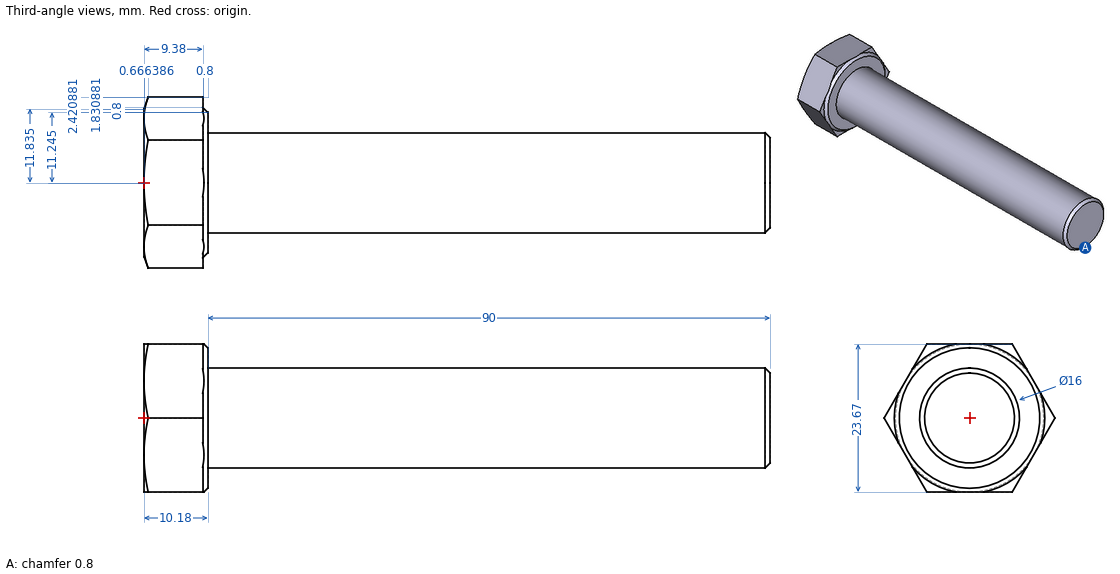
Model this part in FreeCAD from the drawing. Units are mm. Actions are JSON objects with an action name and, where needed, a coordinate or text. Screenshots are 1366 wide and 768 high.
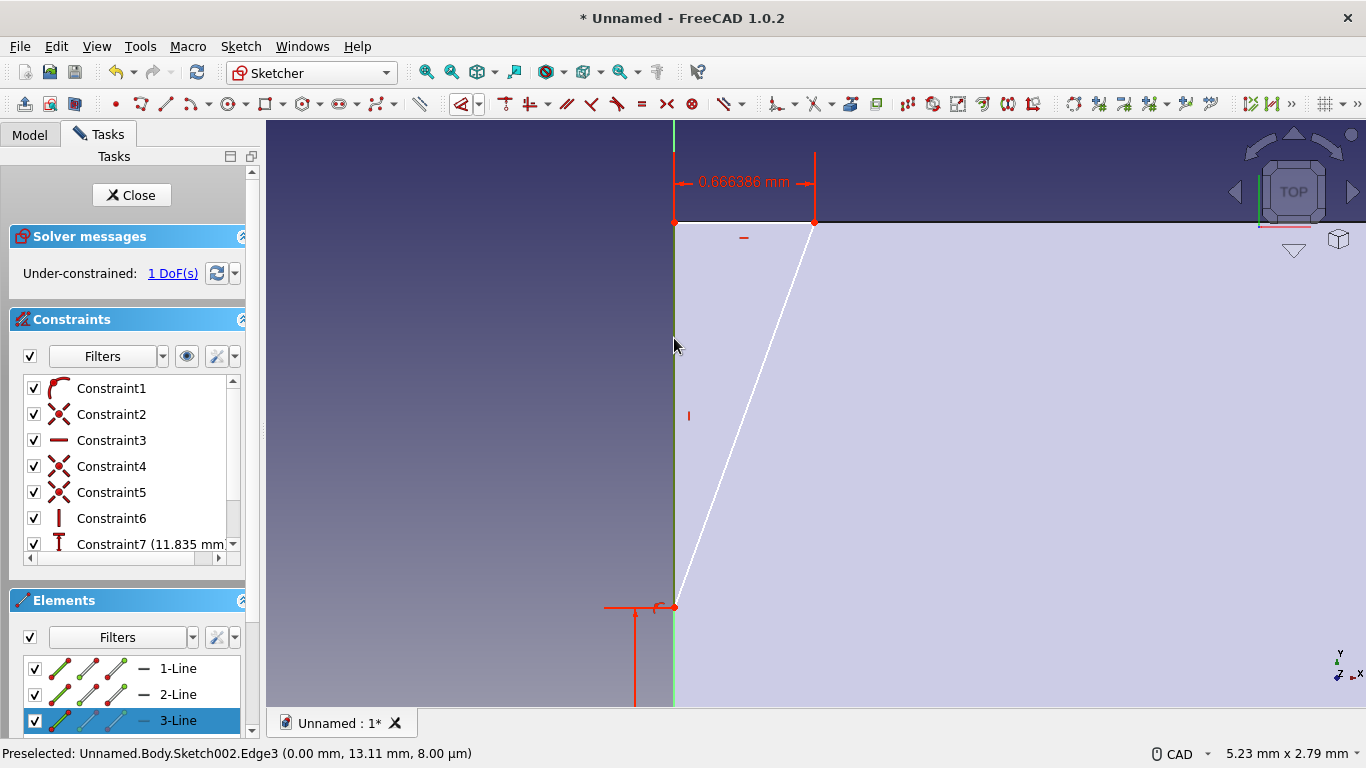
{"action": "key", "text": "i"}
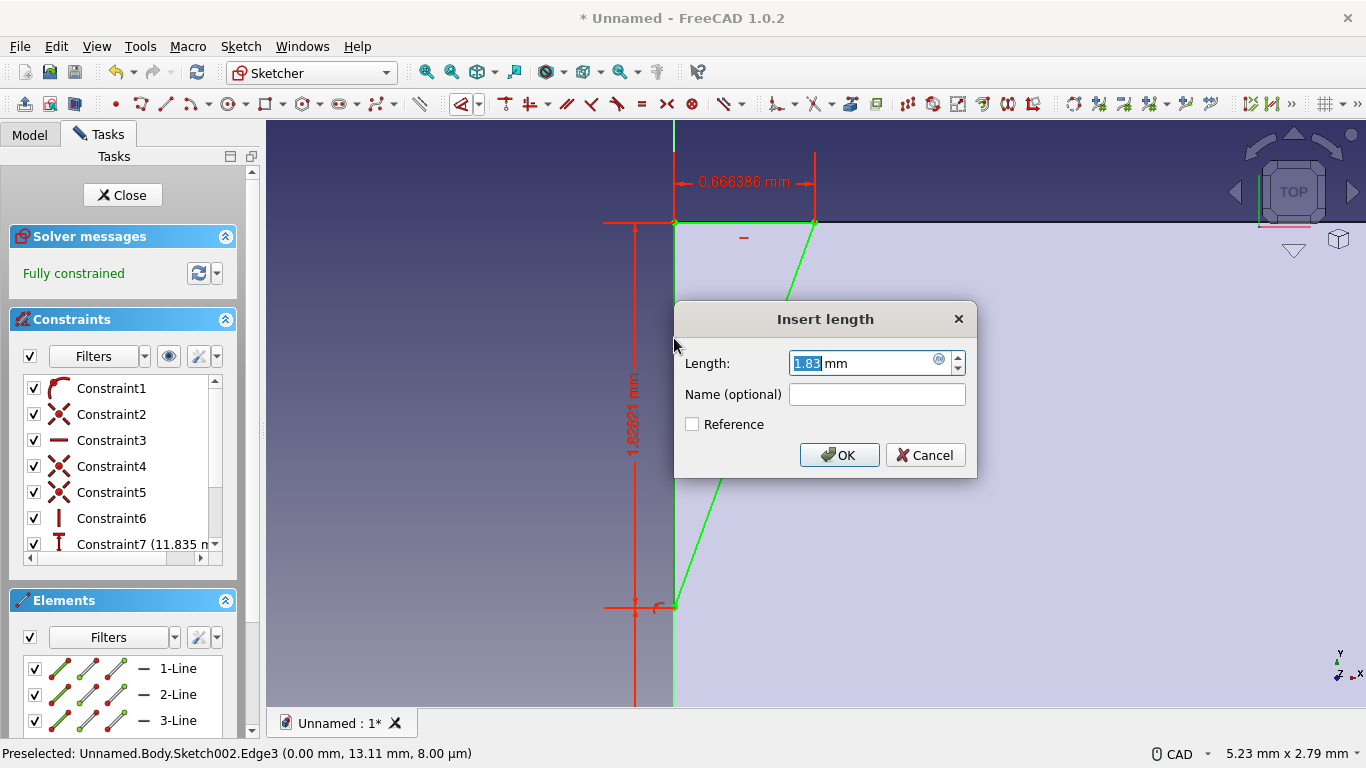
{"action": "type", "text": "1.830881"}
{"action": "key", "text": "Return"}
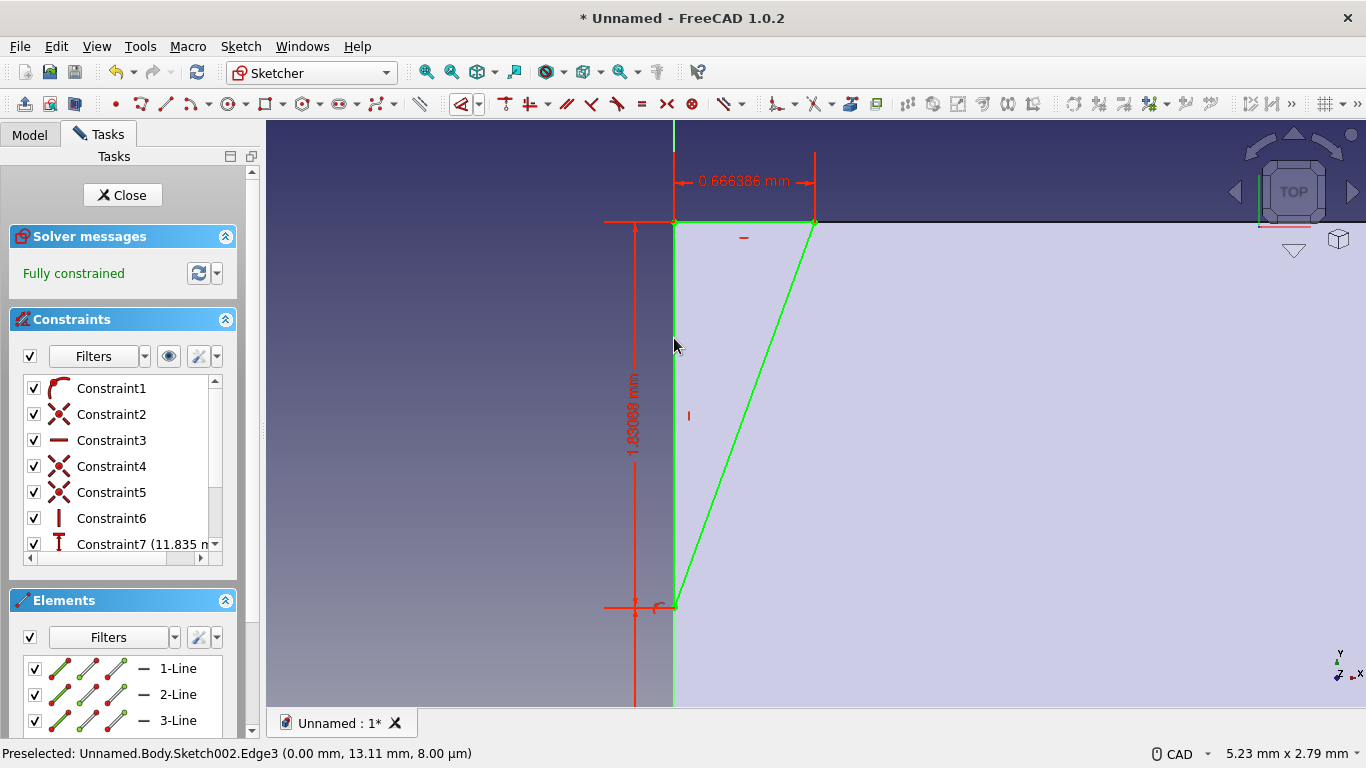
{"action": "left_click", "coordinate": [123, 195]}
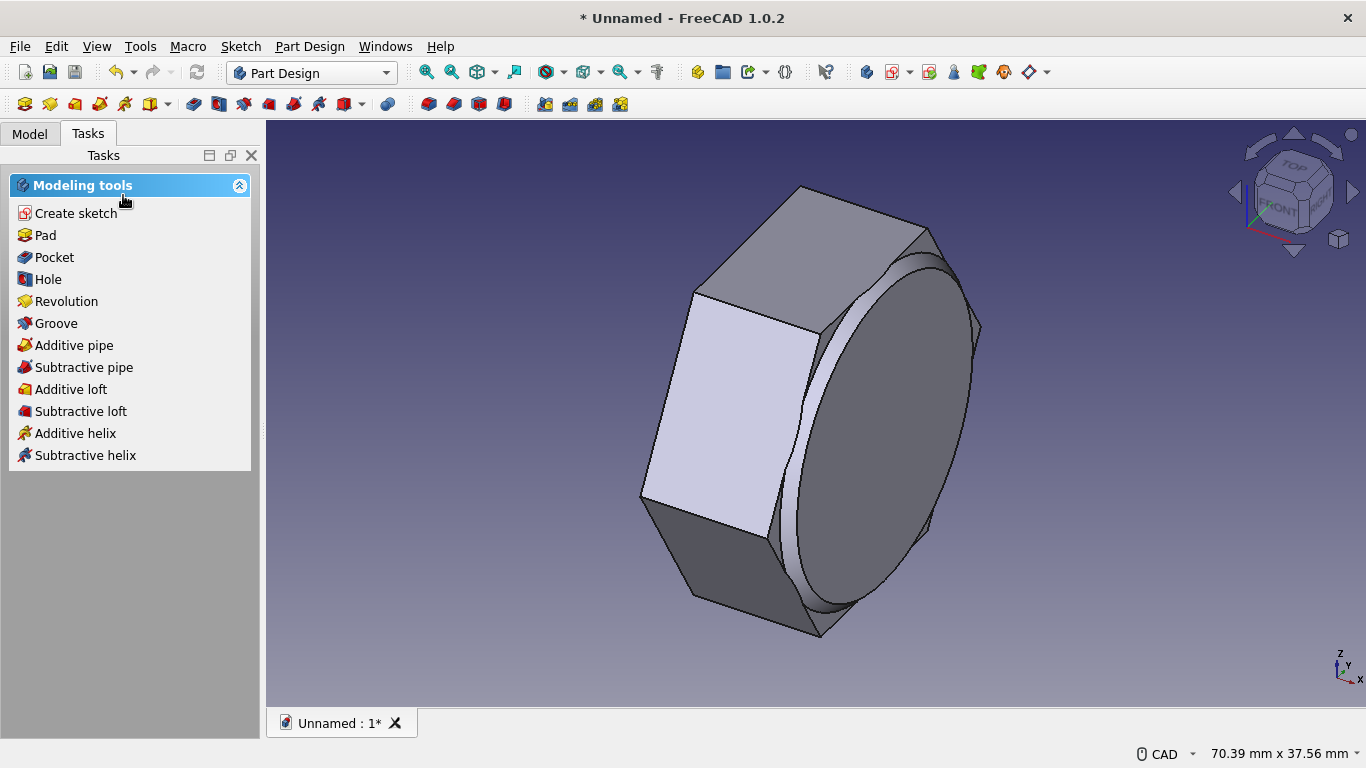
{"action": "left_click", "coordinate": [244, 104]}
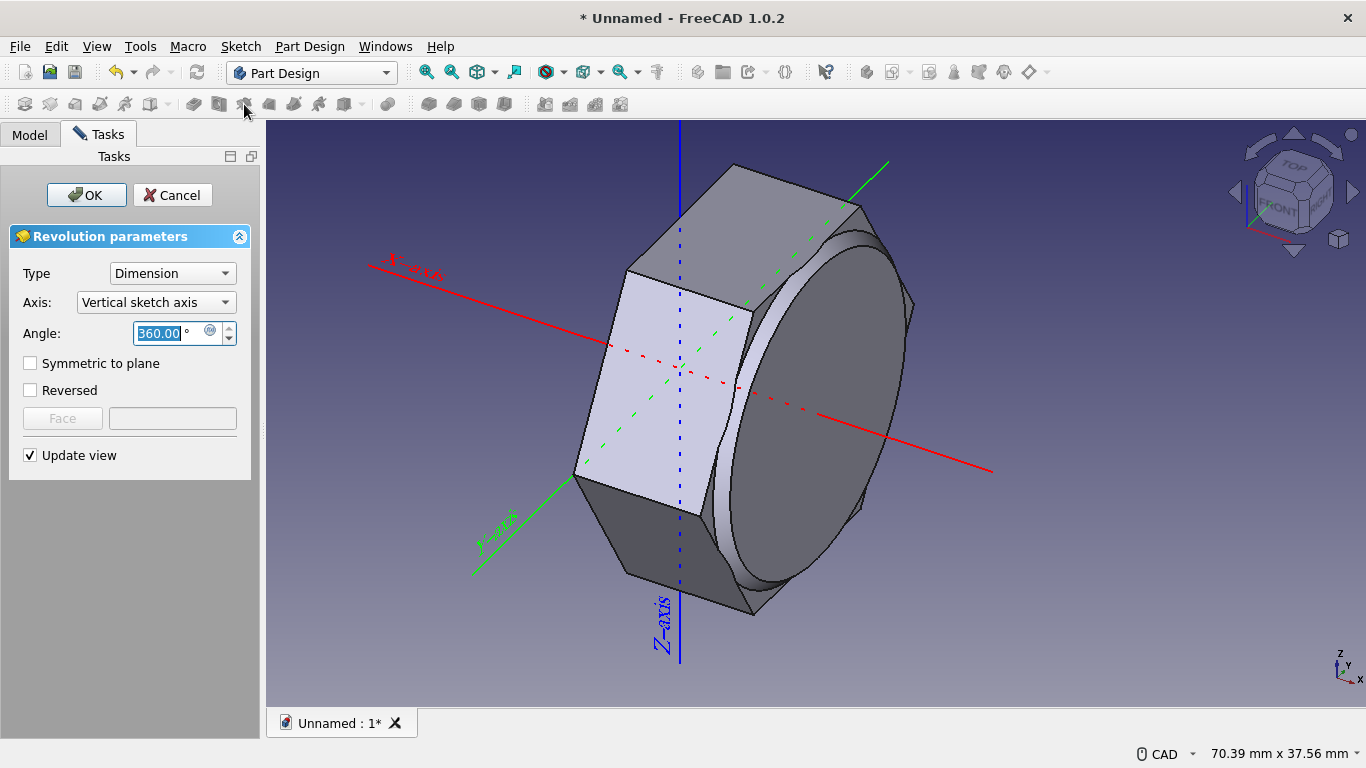
{"action": "left_click", "coordinate": [157, 302]}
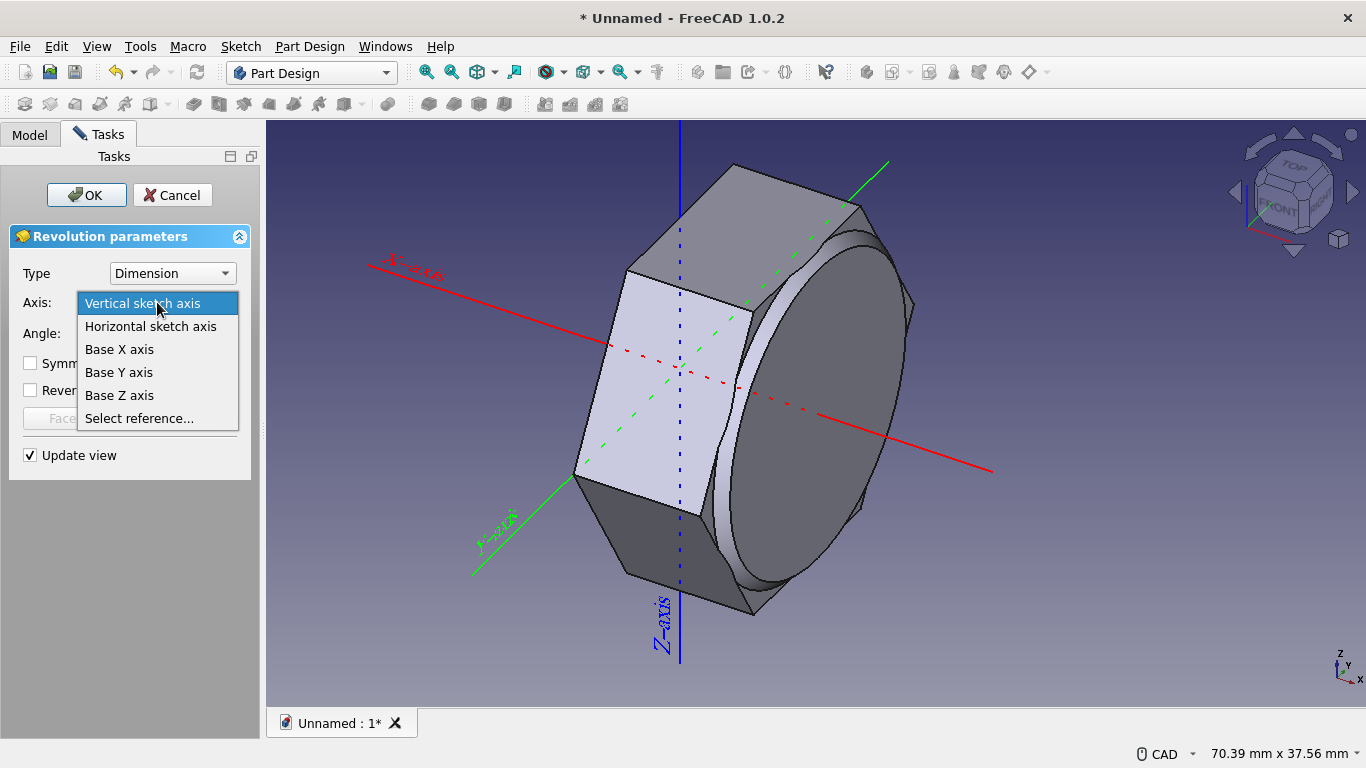
{"action": "left_click", "coordinate": [156, 326]}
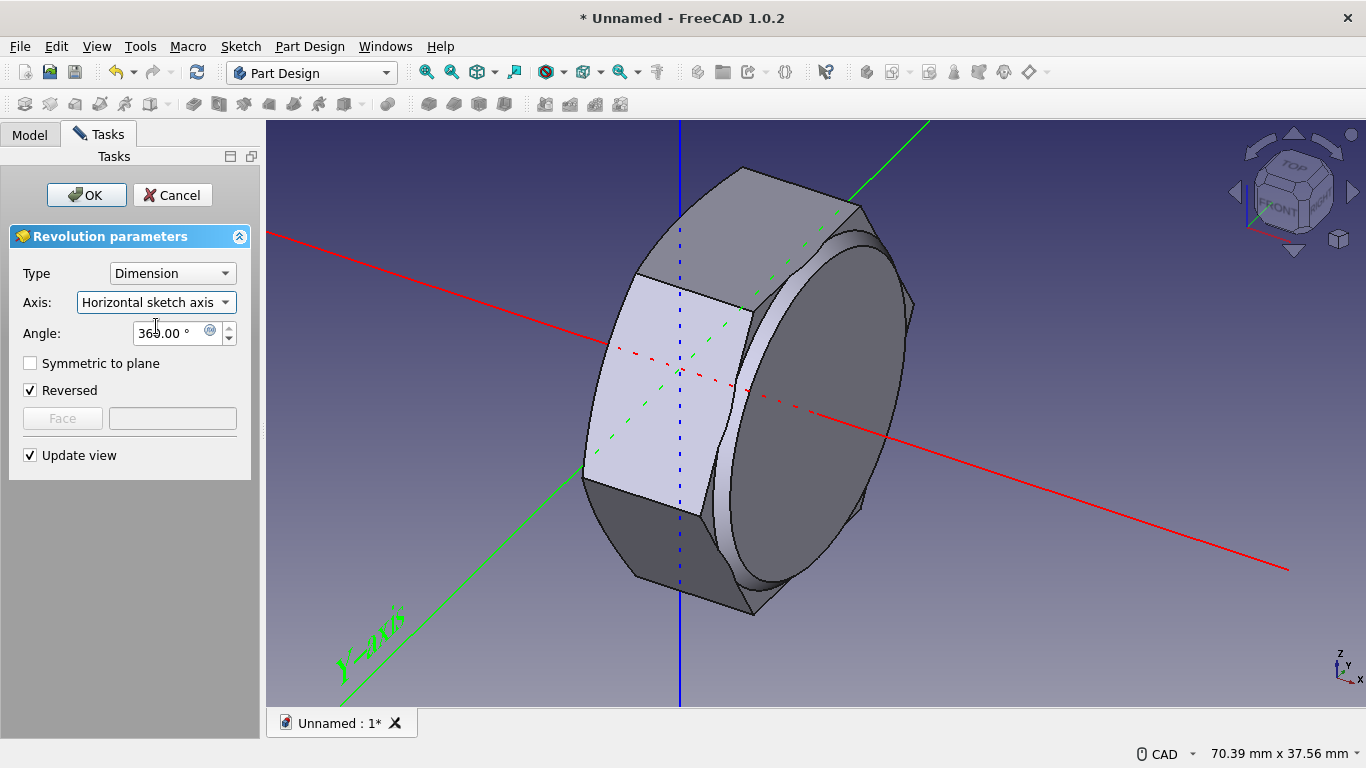
{"action": "left_click", "coordinate": [87, 195]}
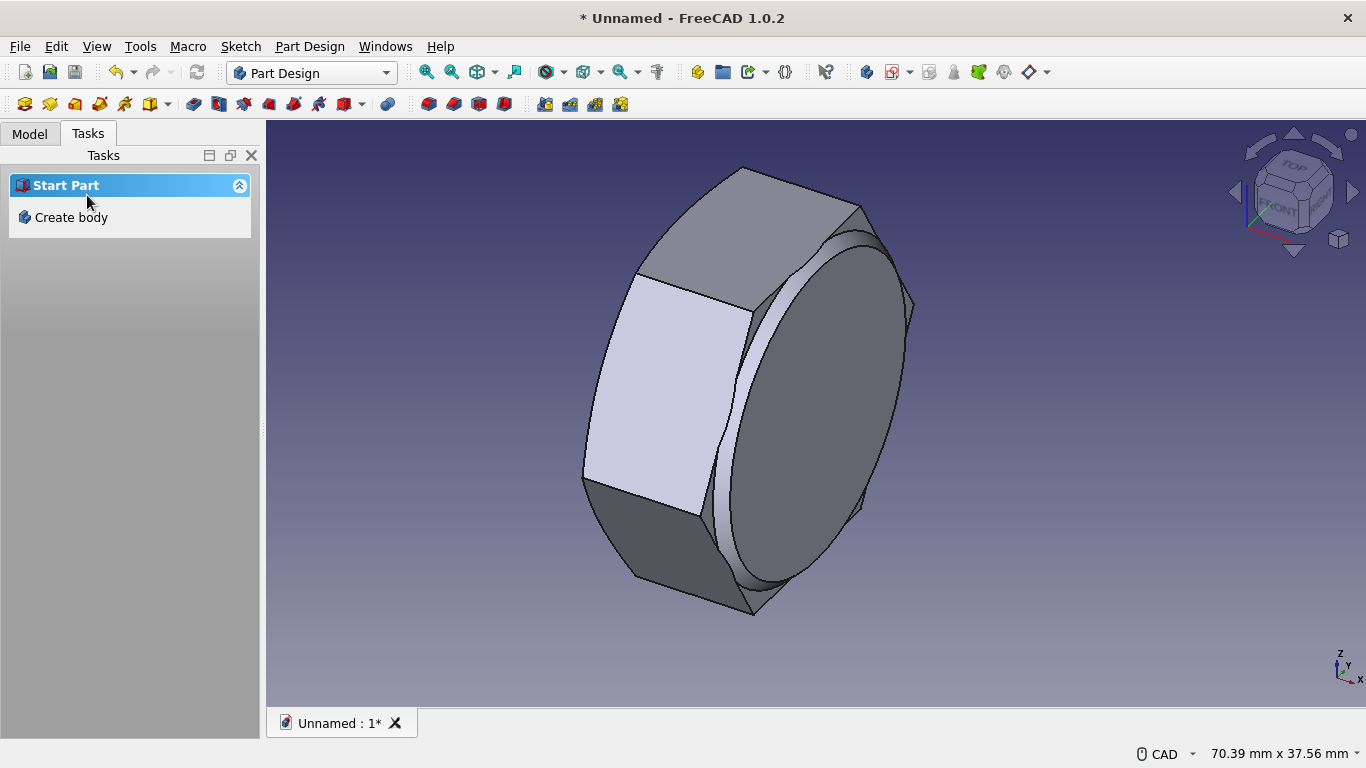
{"action": "key", "text": "v f"}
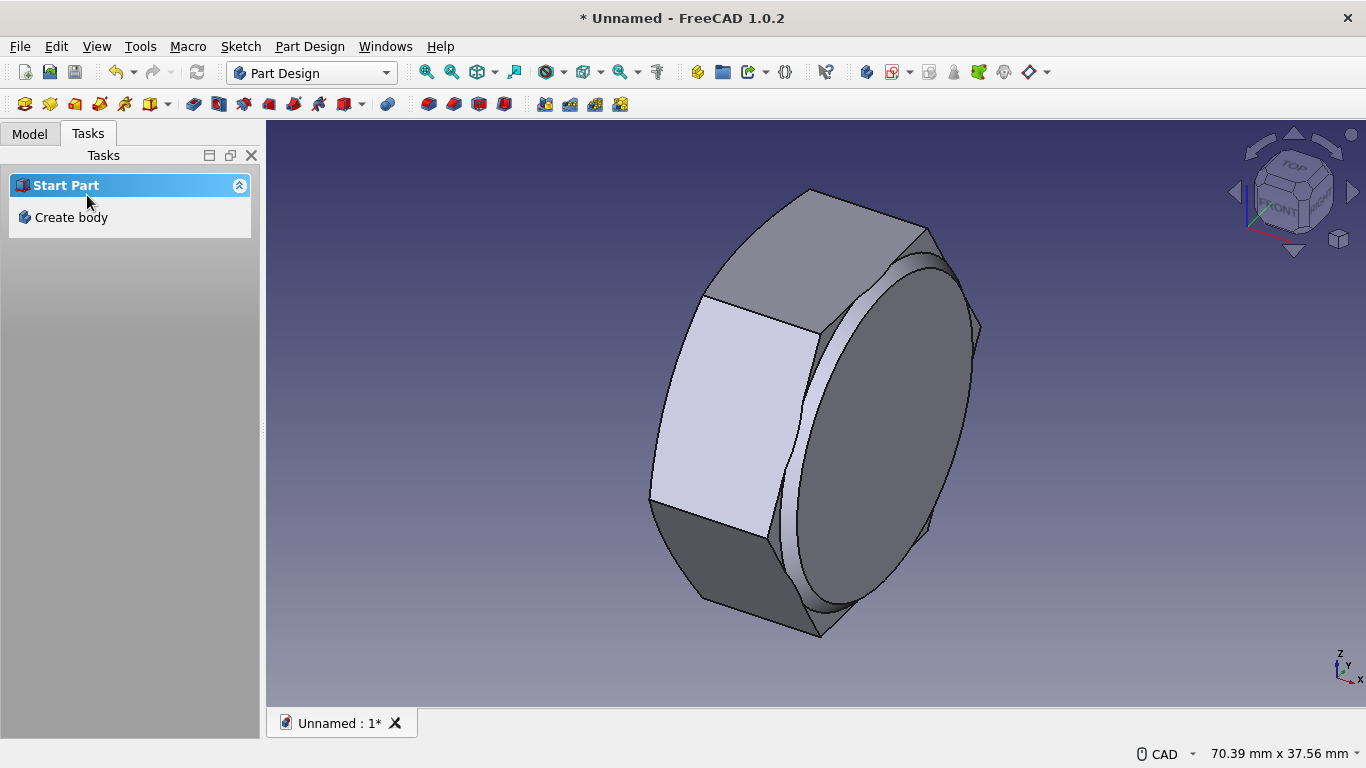
{"action": "left_click", "coordinate": [885, 435]}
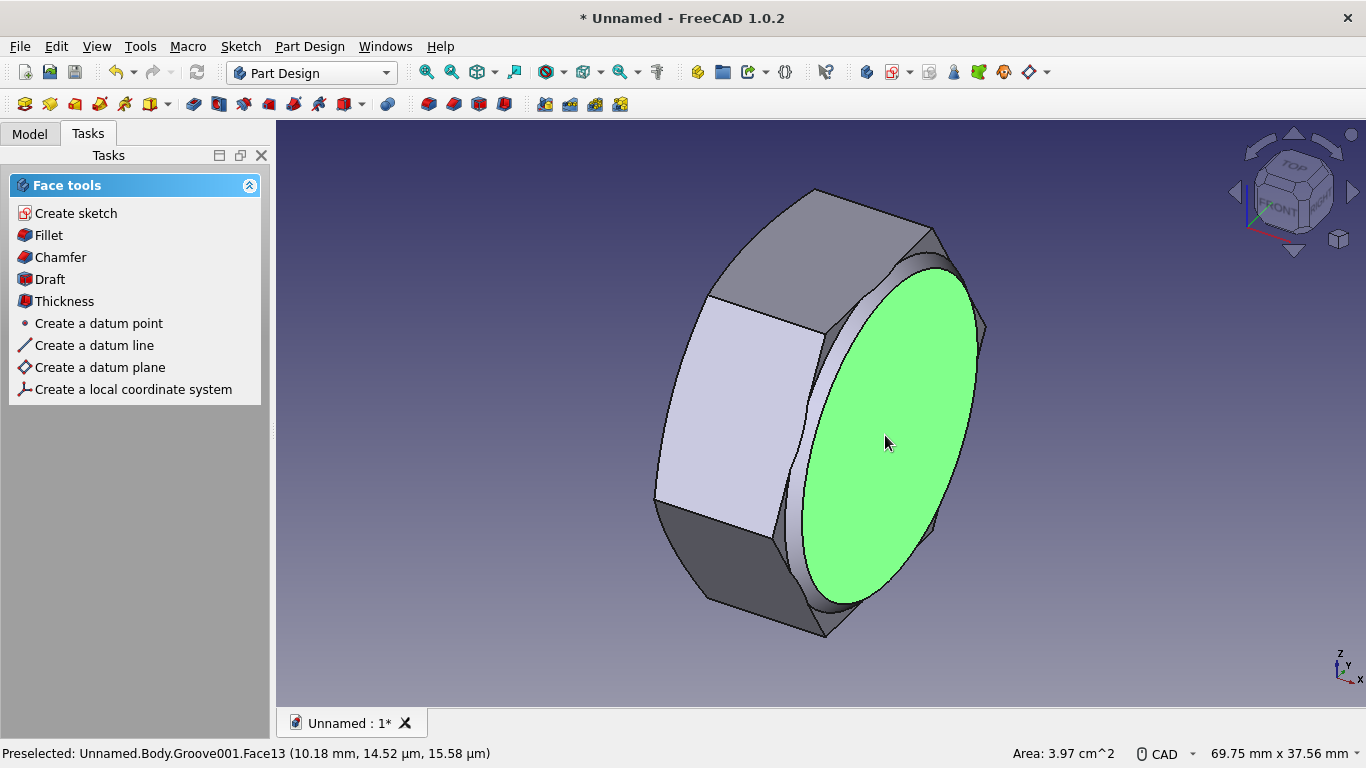
{"action": "left_click", "coordinate": [892, 72]}